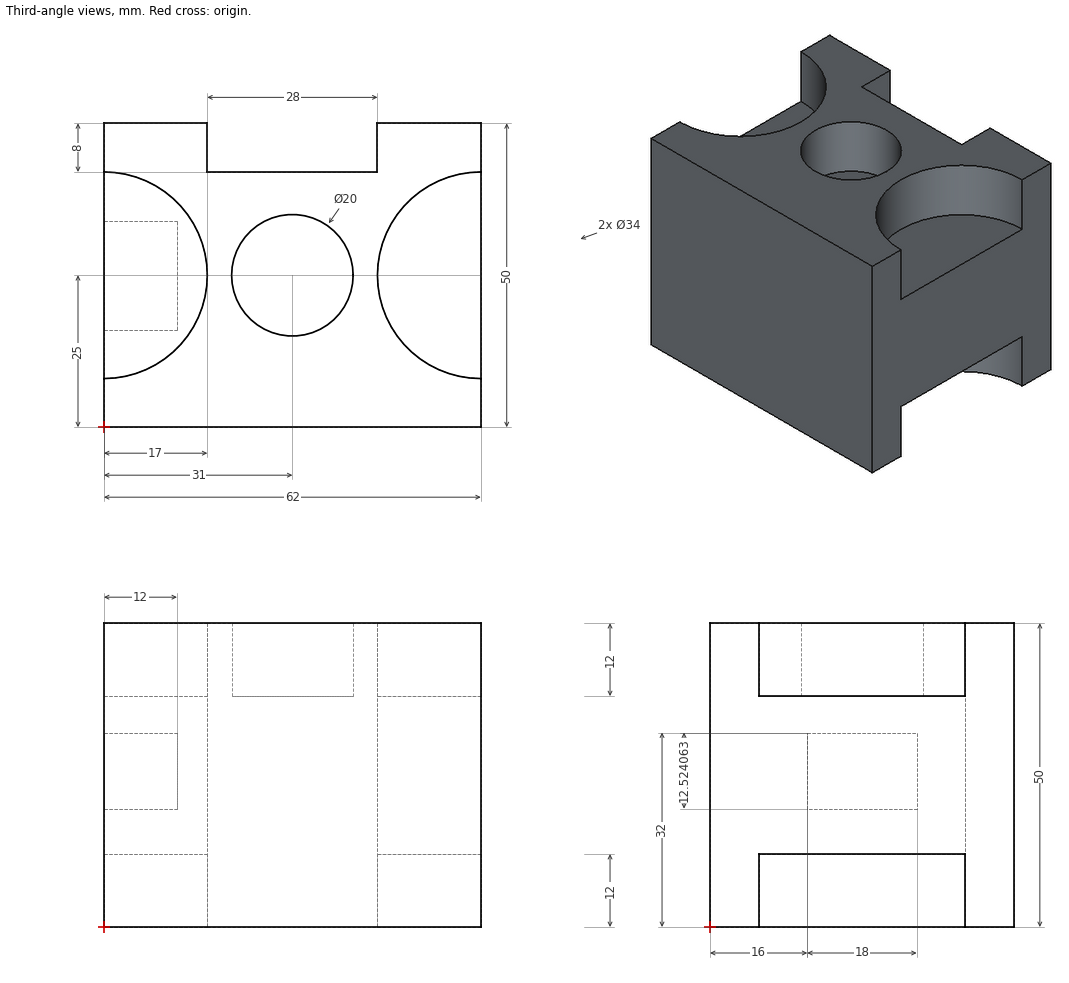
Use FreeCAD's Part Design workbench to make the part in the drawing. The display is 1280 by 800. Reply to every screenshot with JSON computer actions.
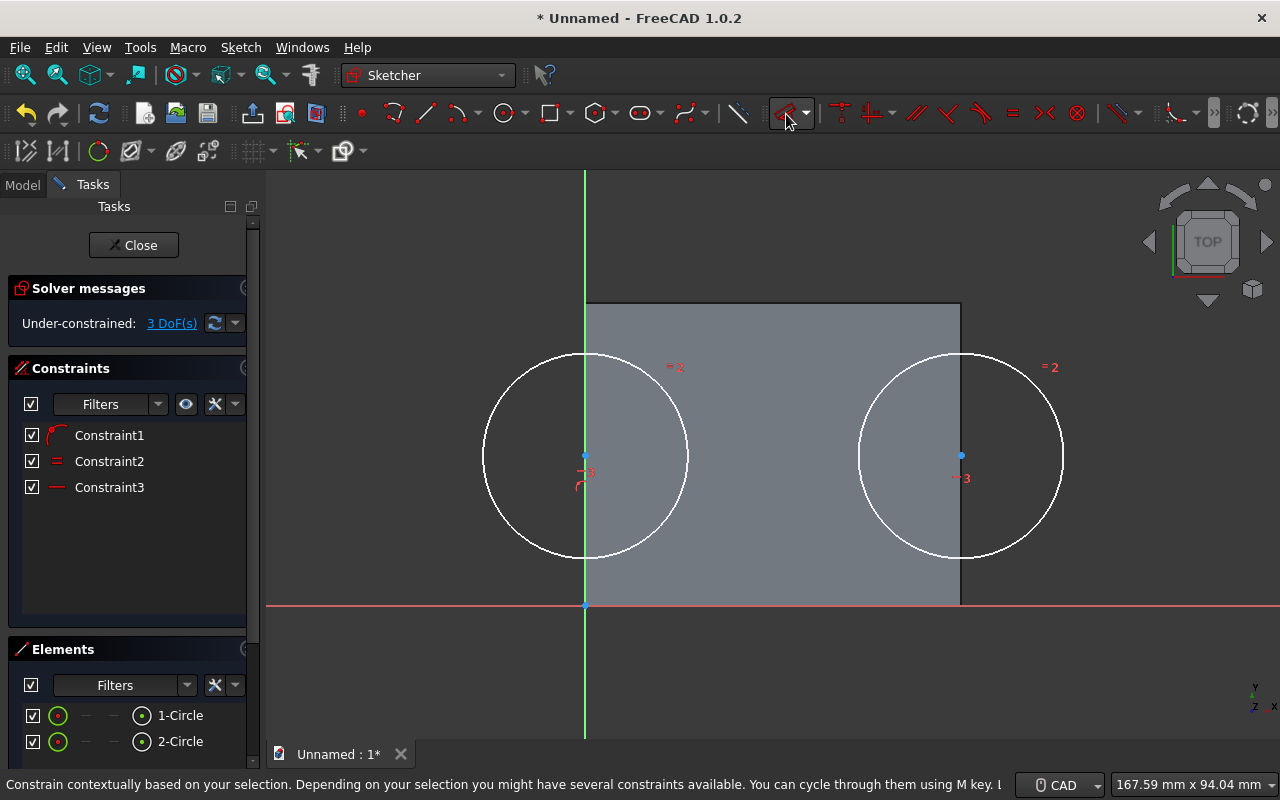
{"action": "left_click", "coordinate": [1033, 383]}
{"action": "left_click", "coordinate": [1055, 360]}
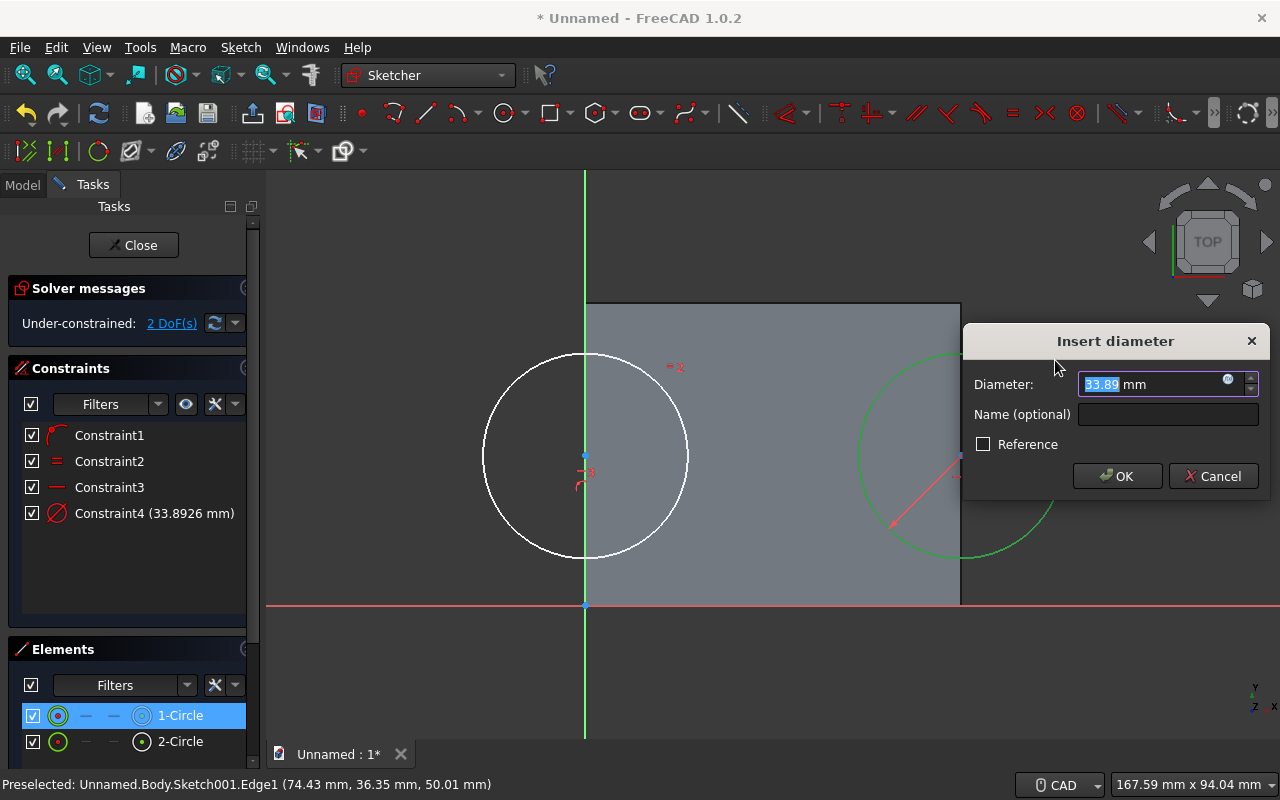
{"action": "type", "text": "34"}
{"action": "key", "text": "Return"}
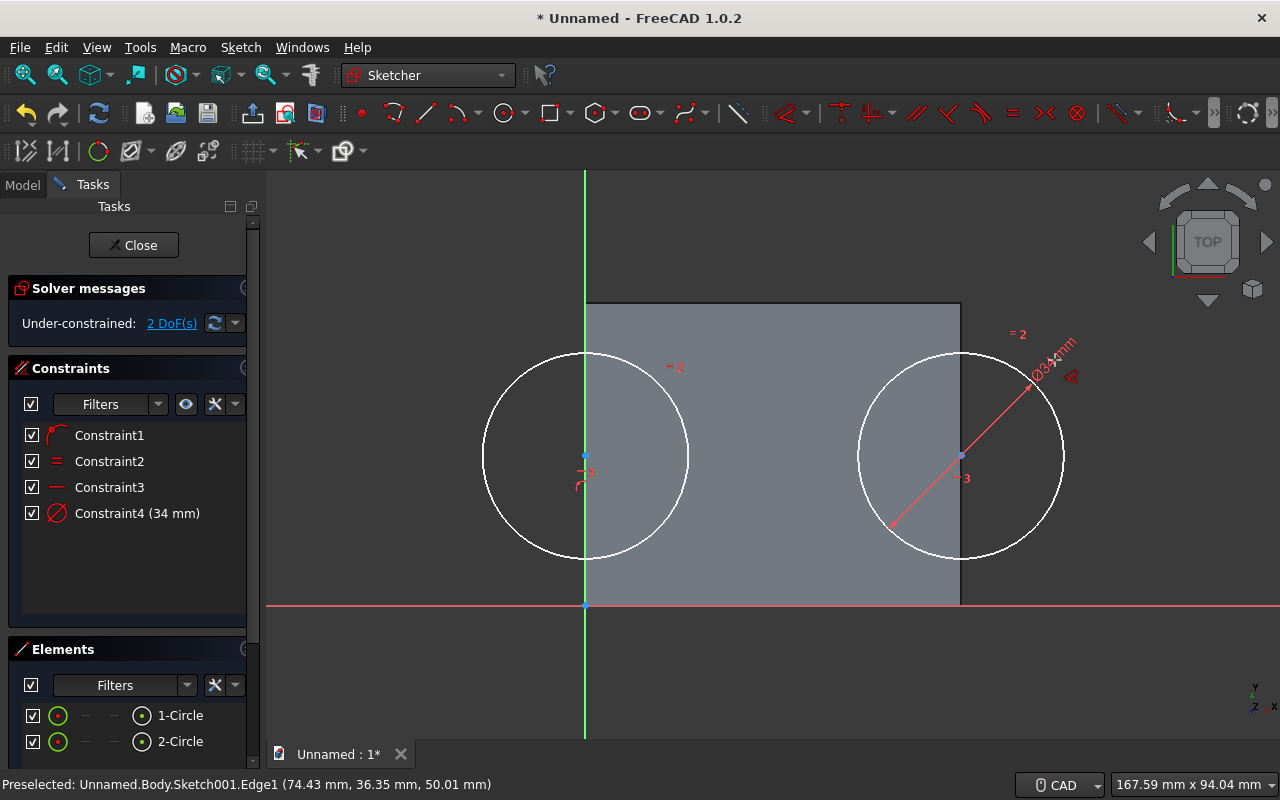
{"action": "left_click", "coordinate": [961, 456]}
{"action": "left_click", "coordinate": [773, 640]}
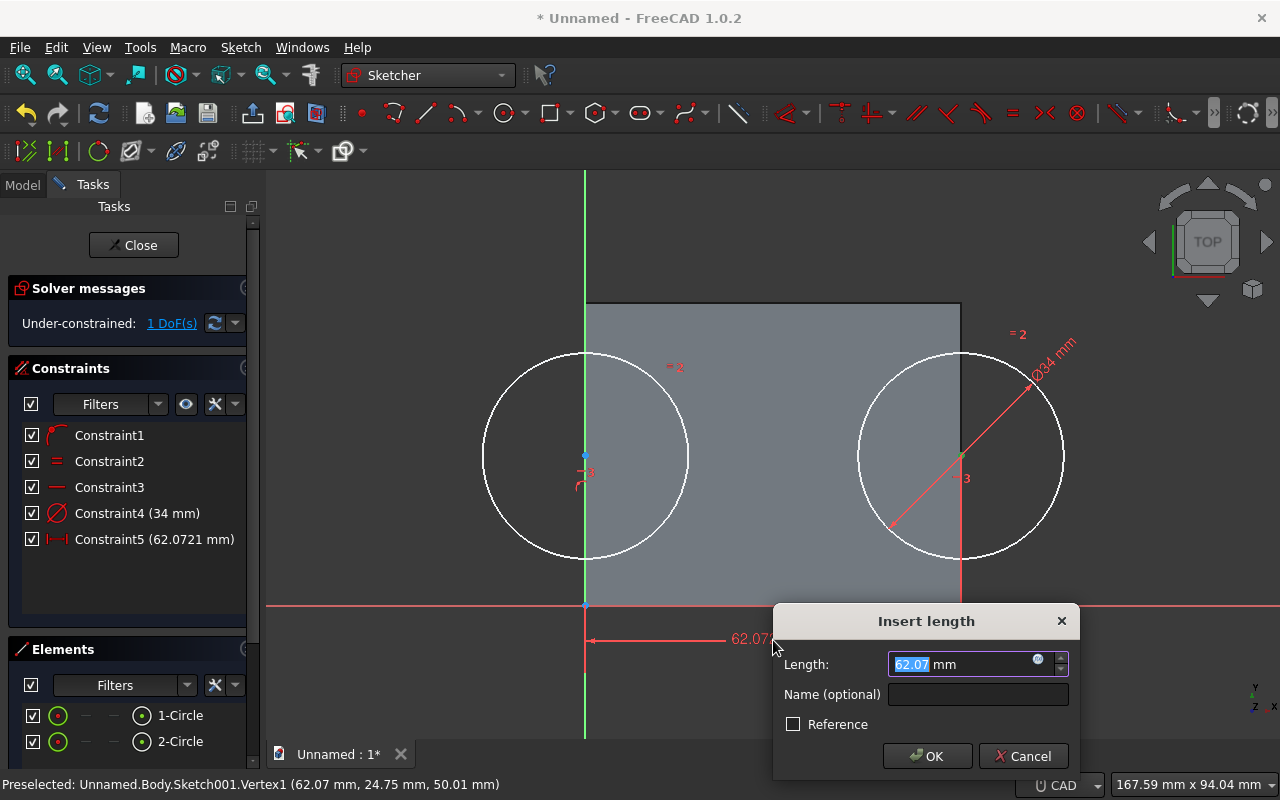
{"action": "type", "text": "62"}
{"action": "key", "text": "Return"}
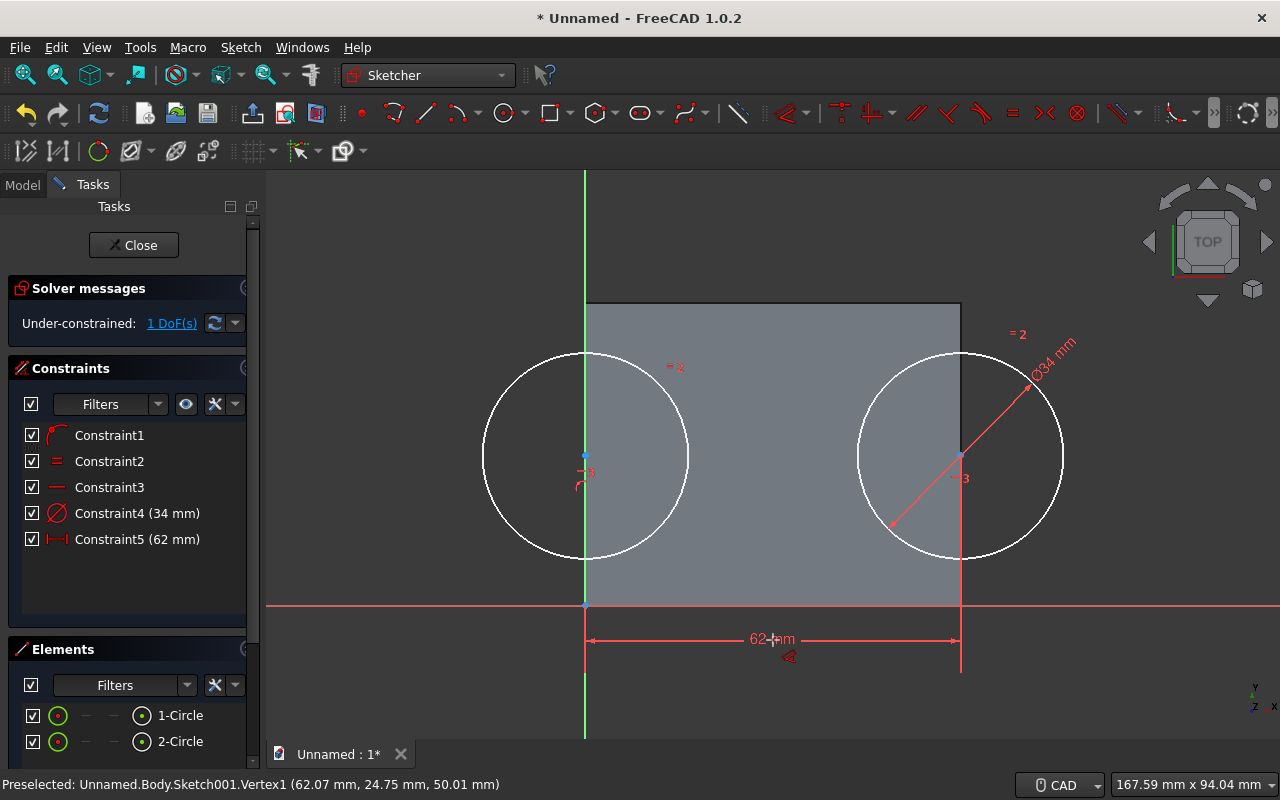
{"action": "left_click", "coordinate": [961, 456]}
{"action": "left_click", "coordinate": [995, 531]}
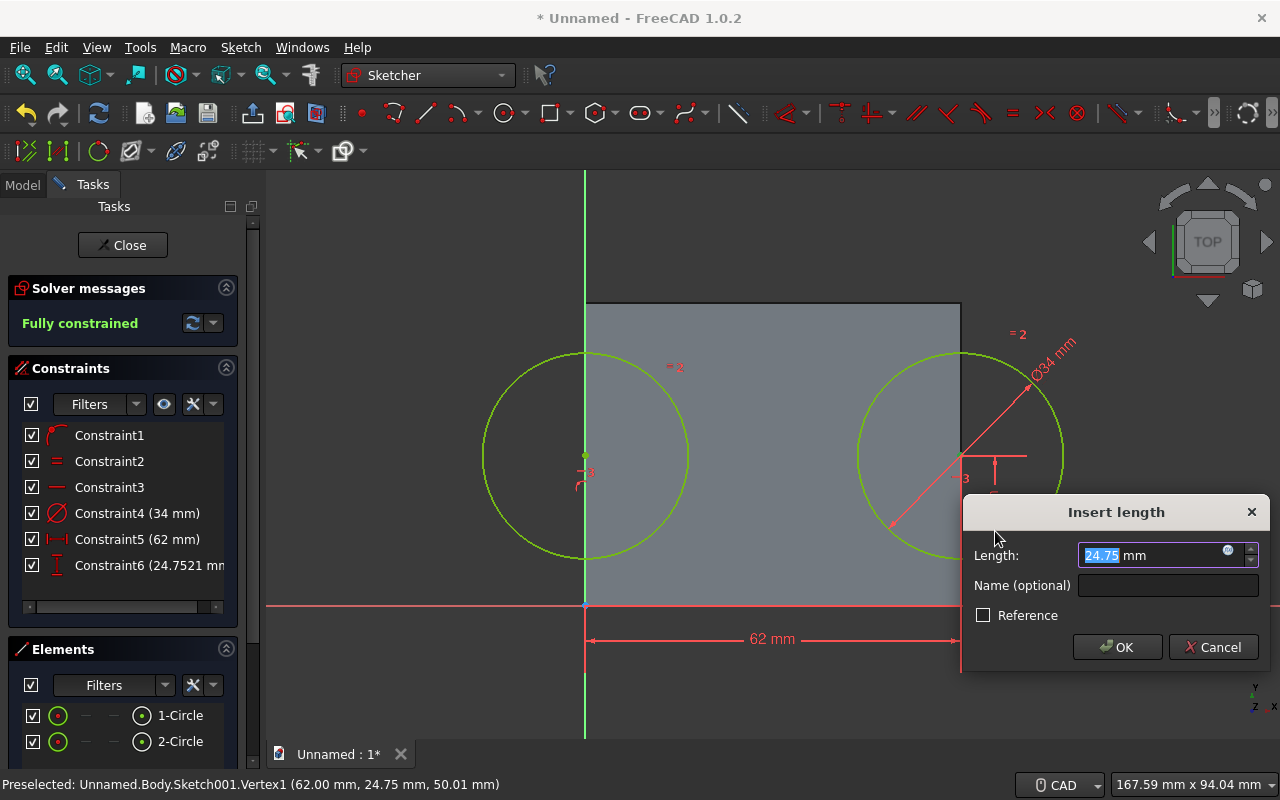
{"action": "type", "text": "25"}
{"action": "key", "text": "Return"}
{"action": "key", "text": "Escape"}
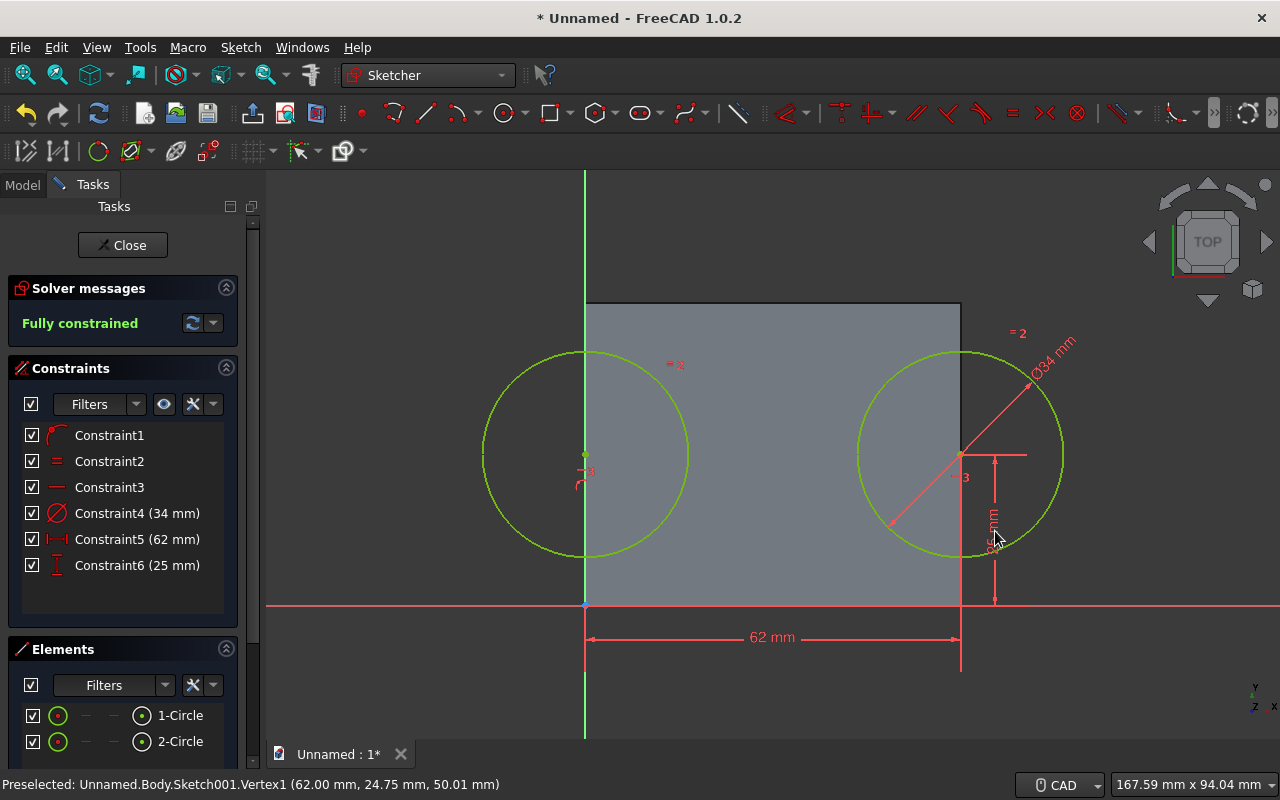
{"action": "left_click", "coordinate": [123, 245]}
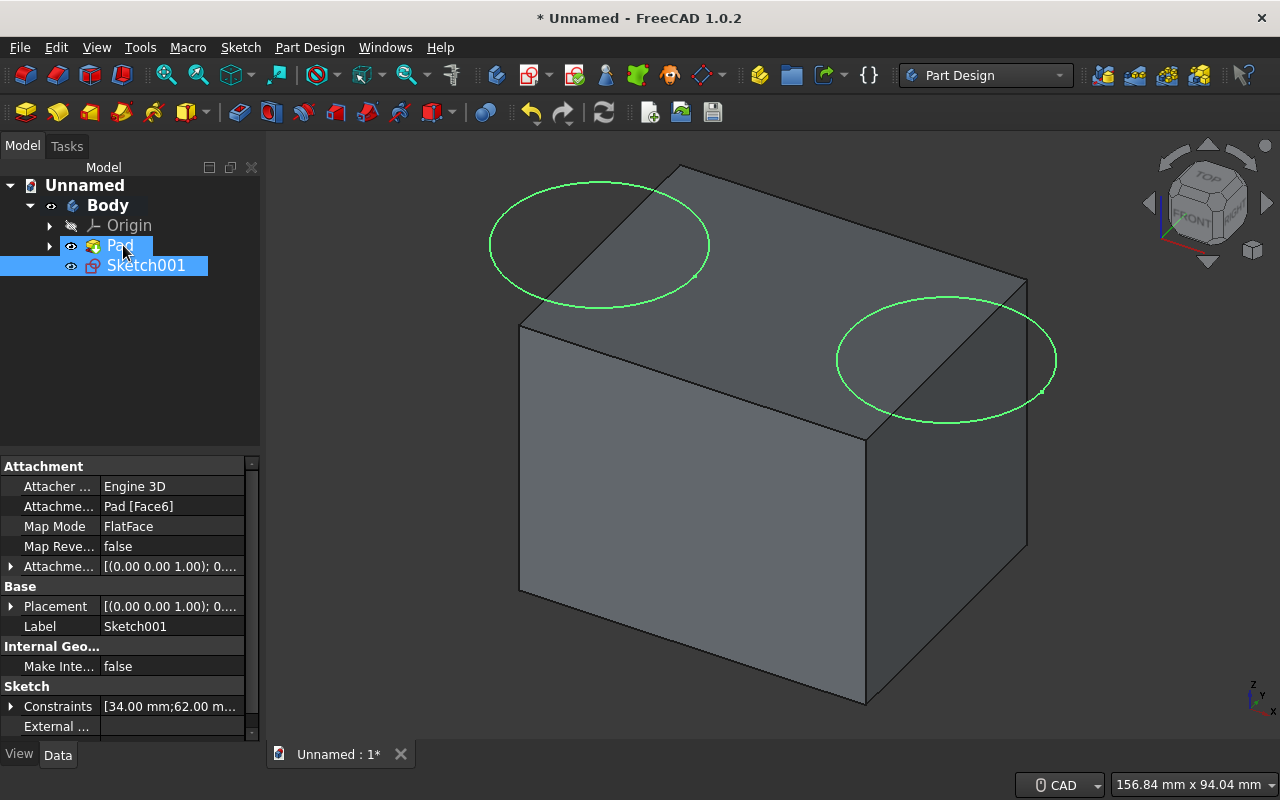
{"action": "left_click", "coordinate": [240, 112]}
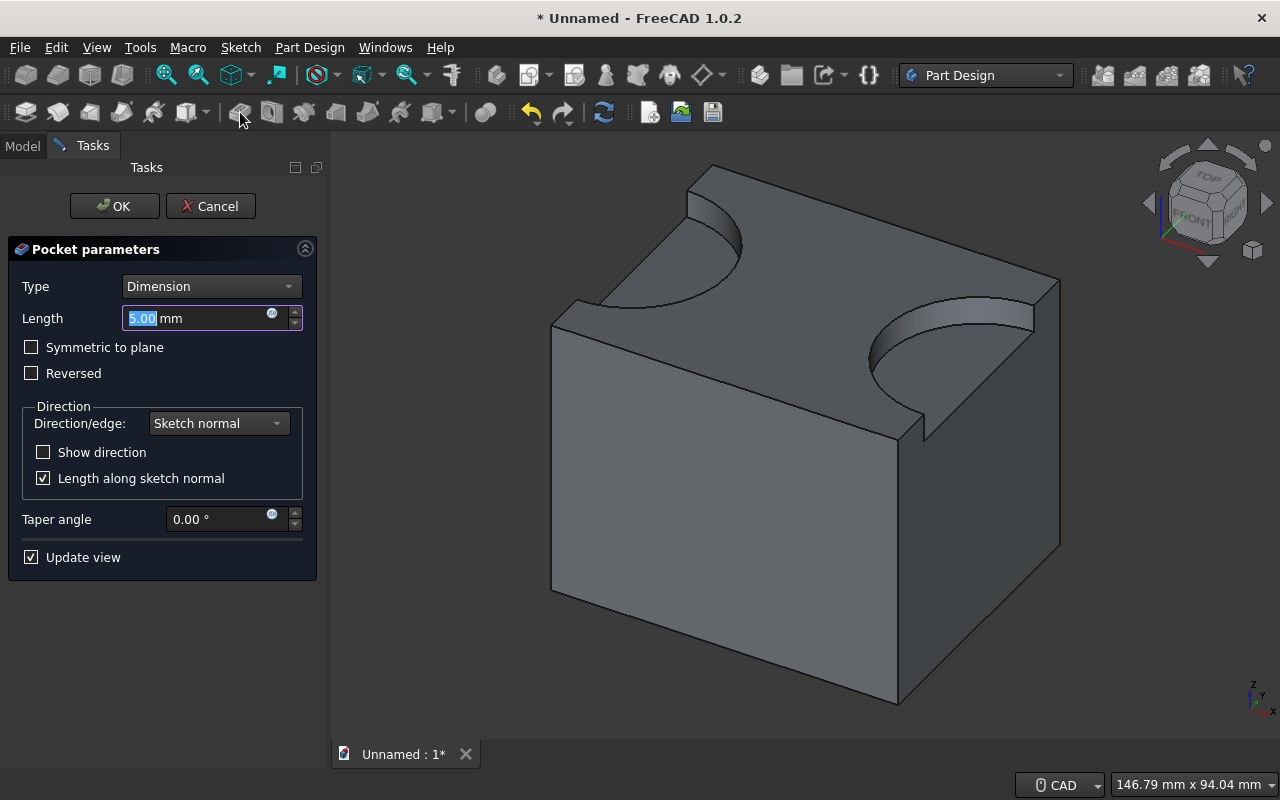
{"action": "type", "text": "12"}
{"action": "key", "text": "Tab"}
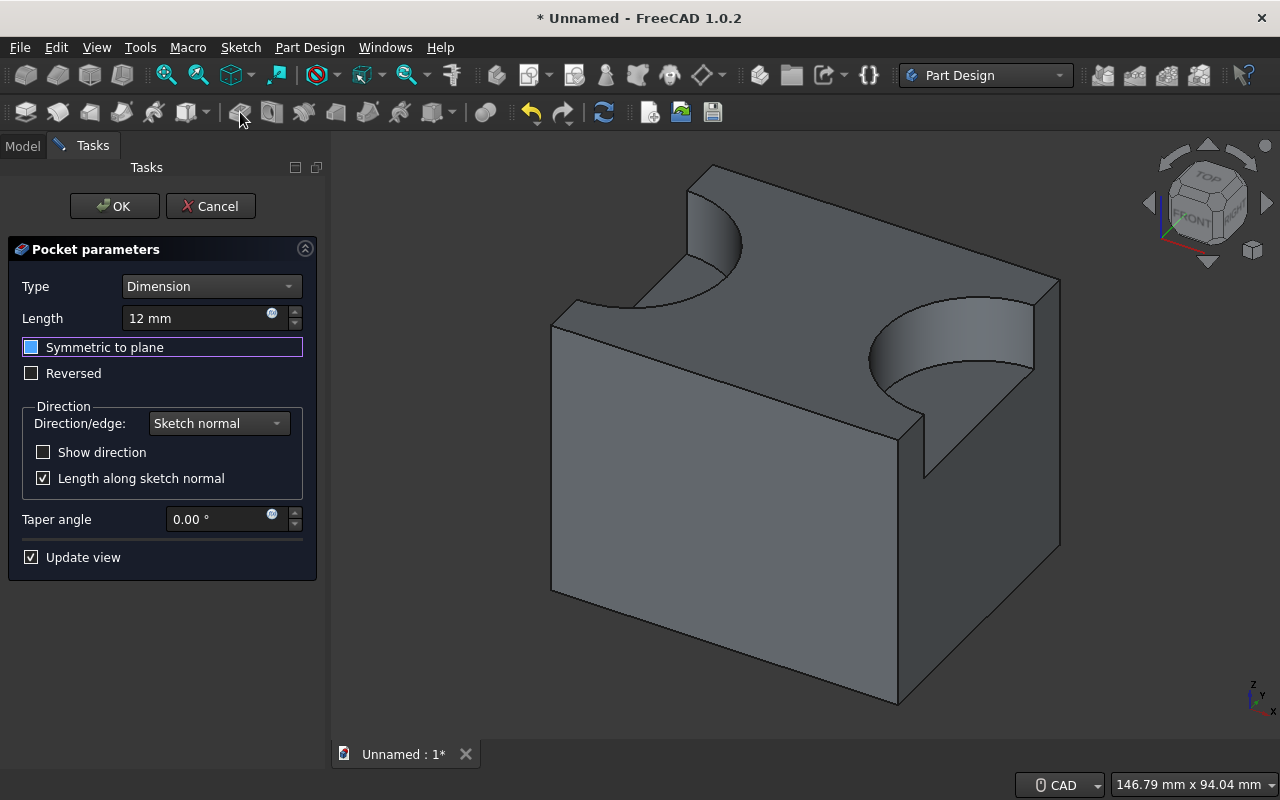
{"action": "left_click", "coordinate": [115, 206]}